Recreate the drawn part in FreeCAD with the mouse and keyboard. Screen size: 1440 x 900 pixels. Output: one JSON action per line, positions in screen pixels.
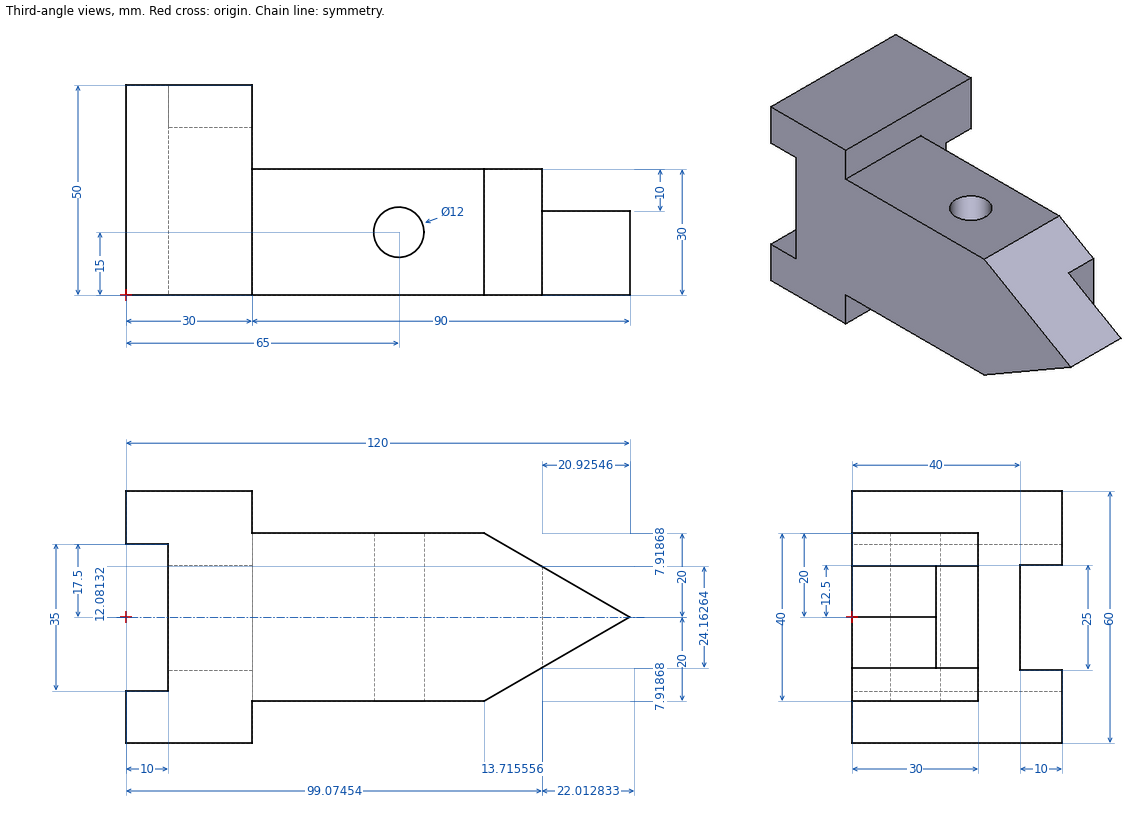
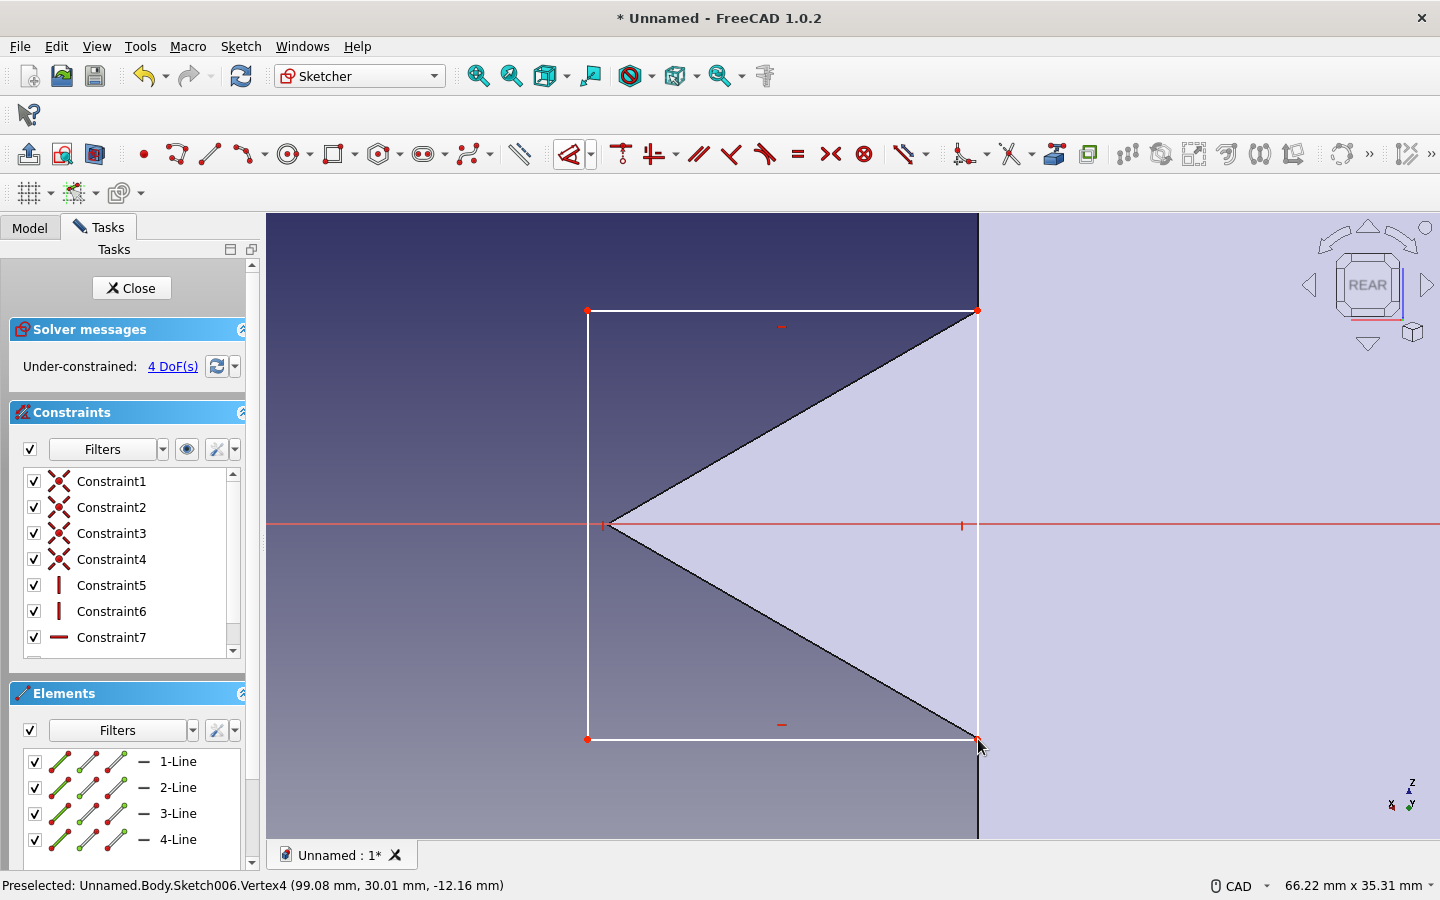
{"action": "left_click", "coordinate": [588, 440]}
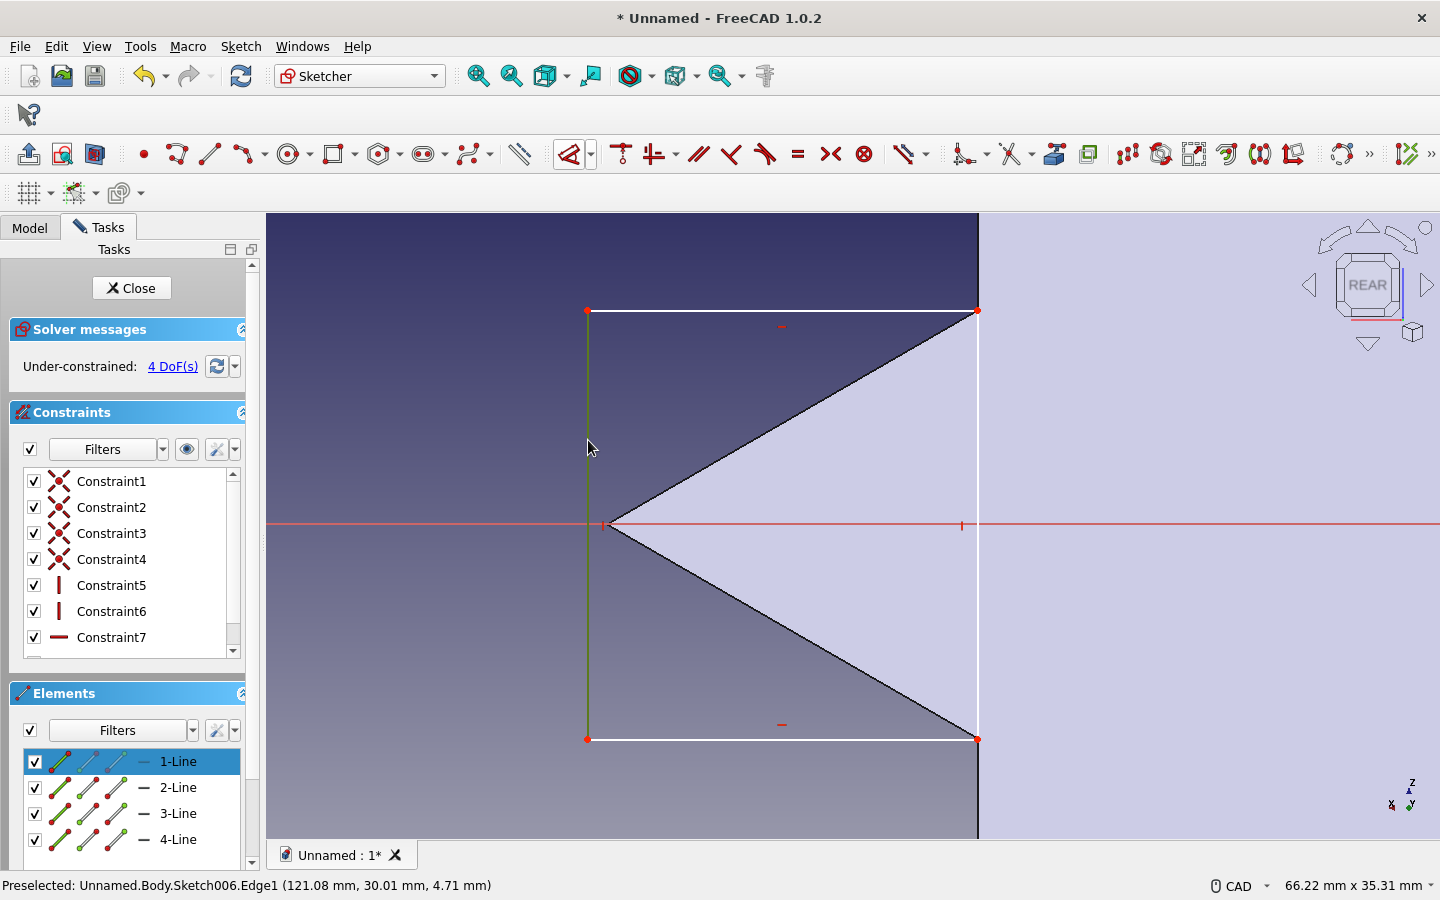
{"action": "left_click", "coordinate": [590, 154]}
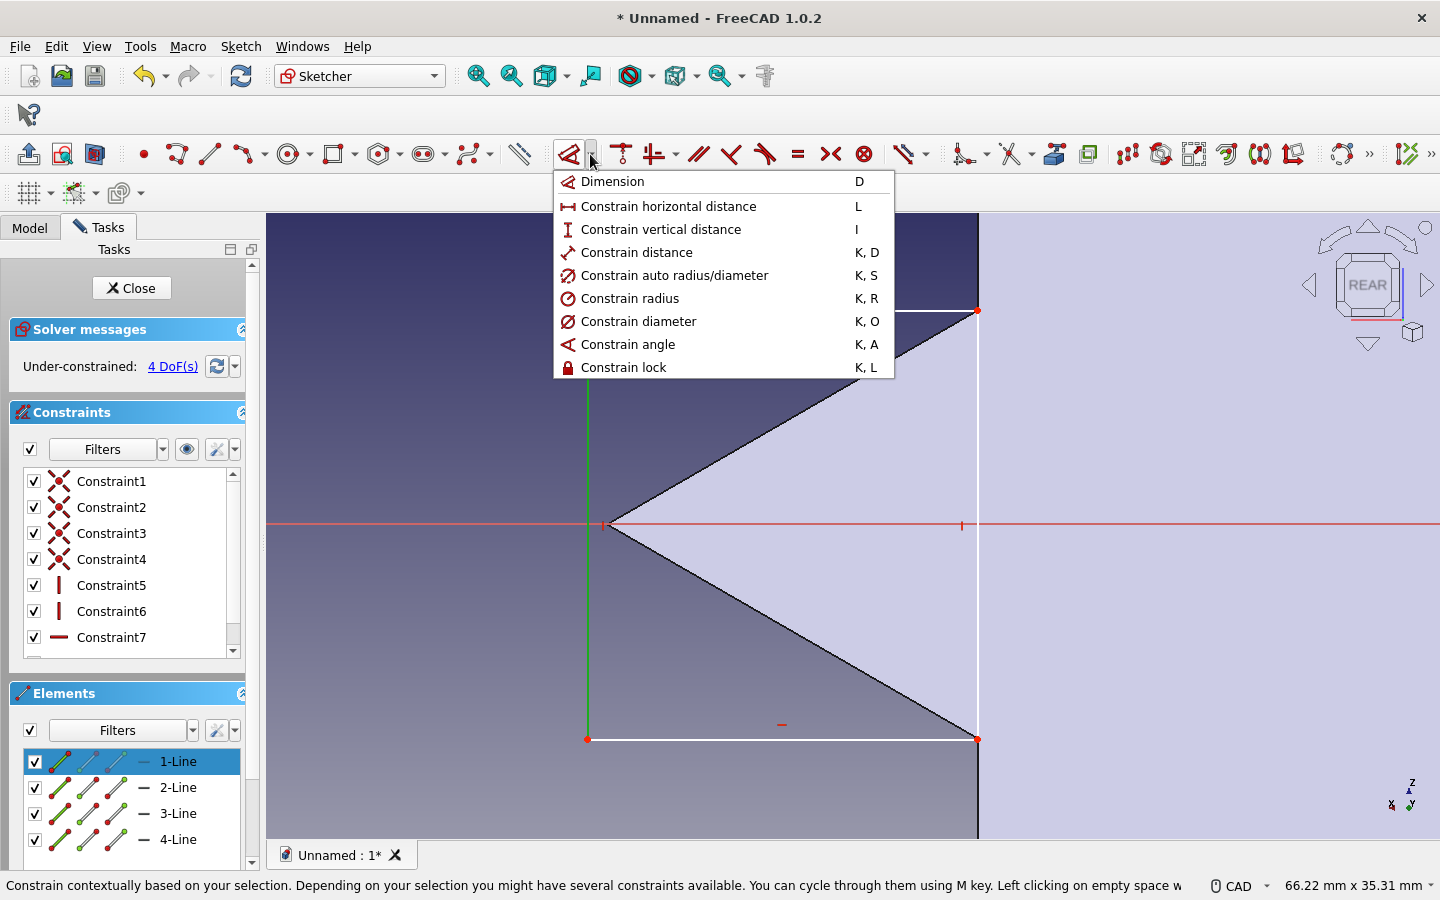
{"action": "left_click", "coordinate": [724, 230]}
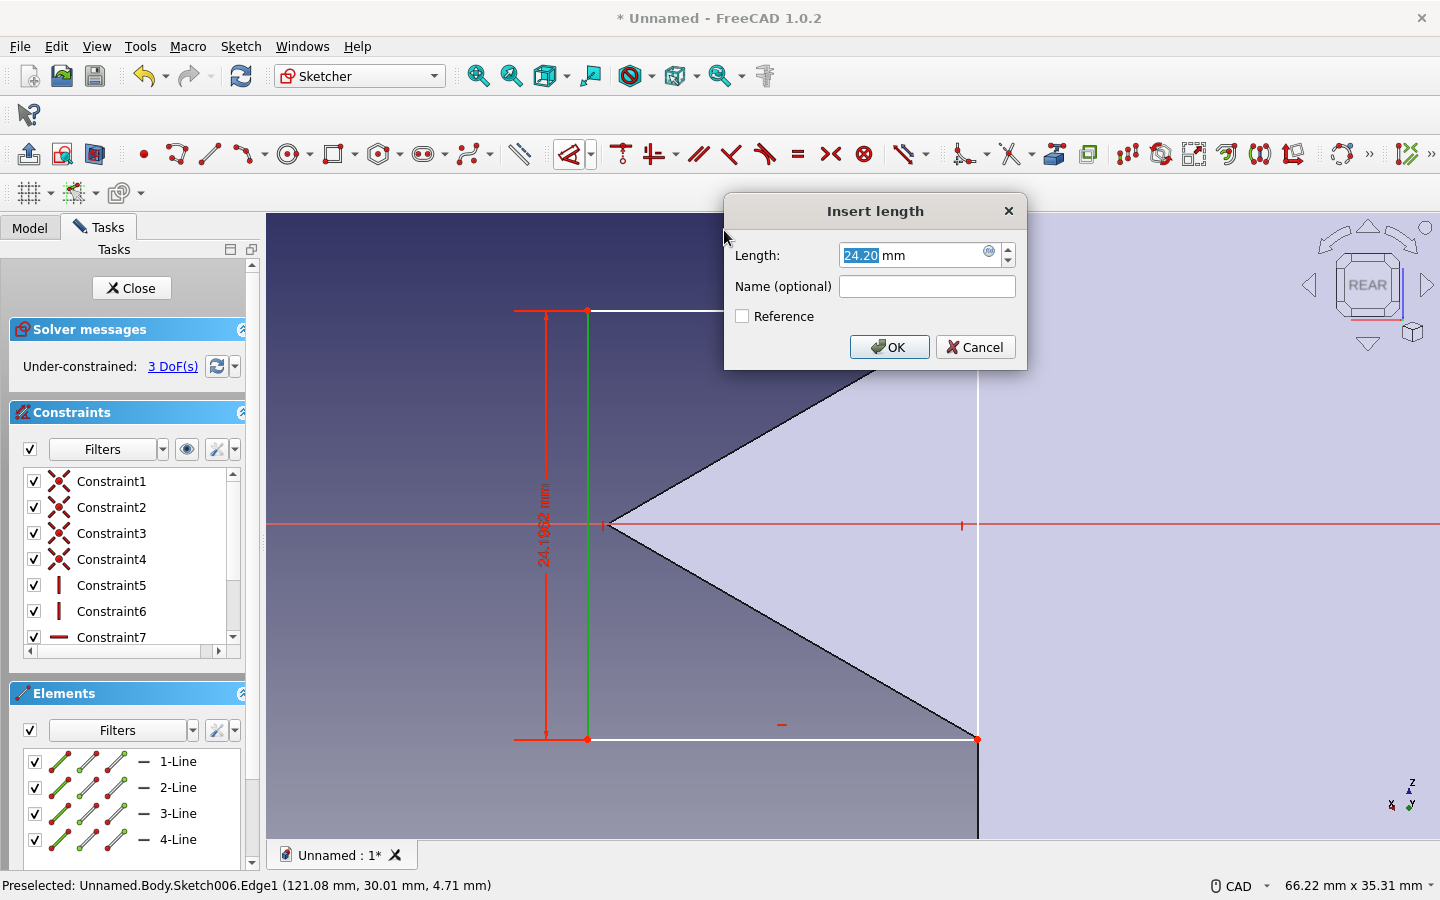
{"action": "type", "text": "24.16264"}
{"action": "key", "text": "Return"}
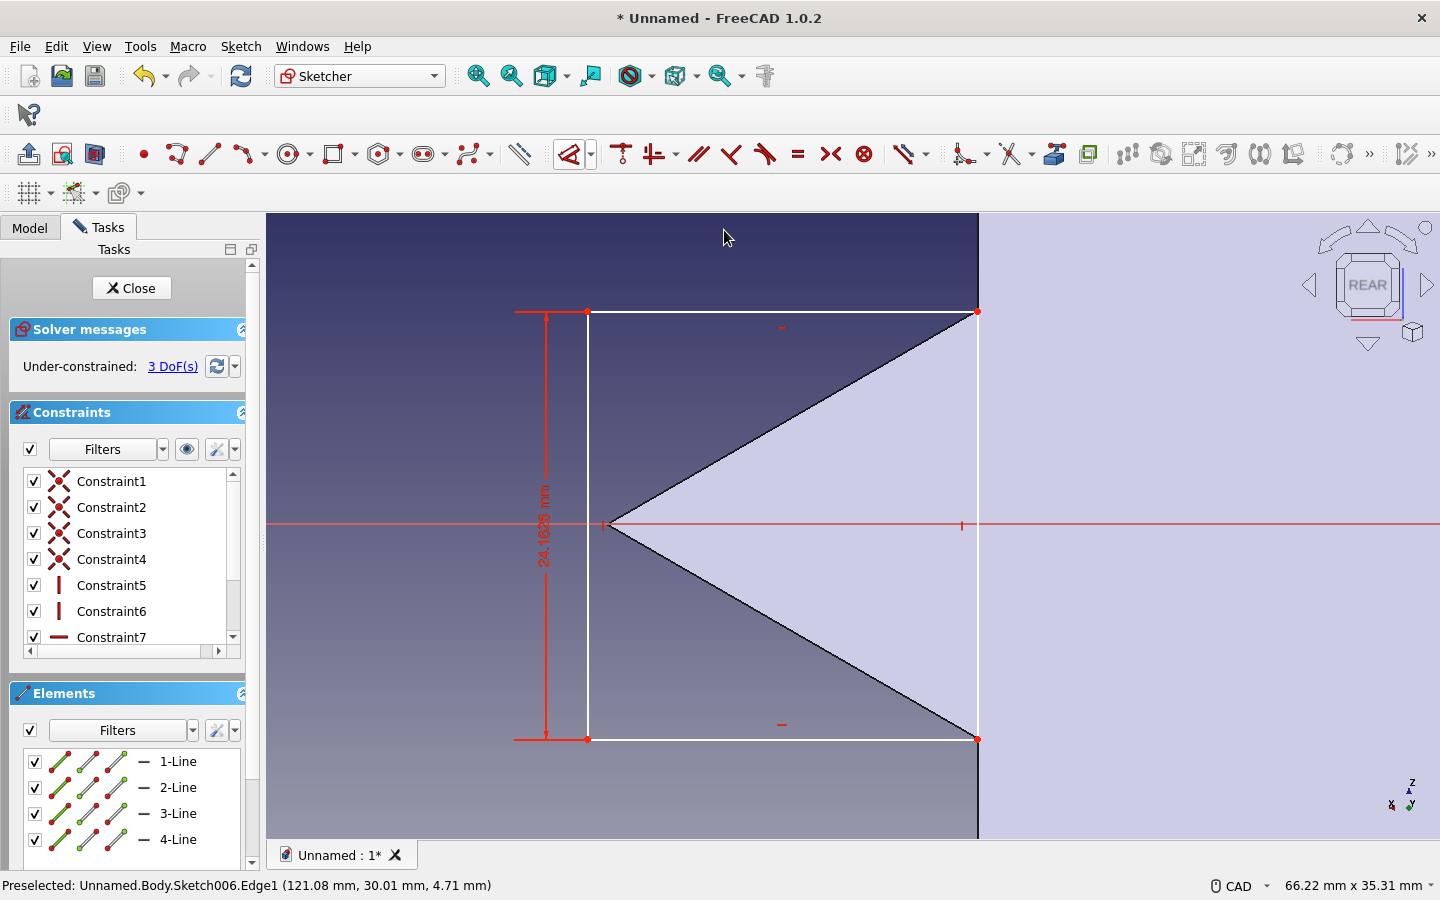
{"action": "left_click", "coordinate": [705, 740]}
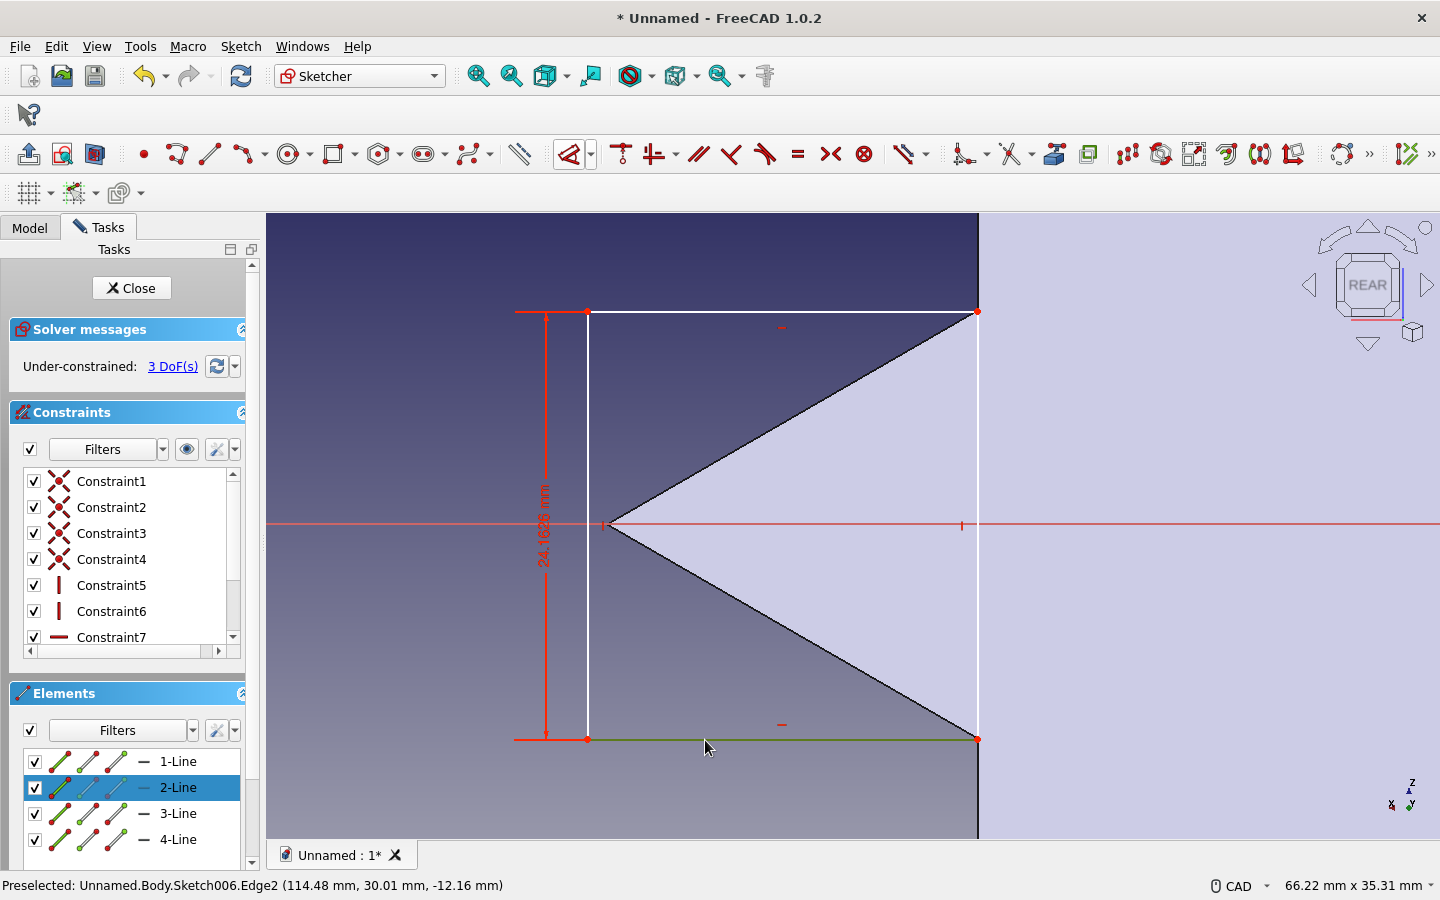
{"action": "left_click", "coordinate": [590, 154]}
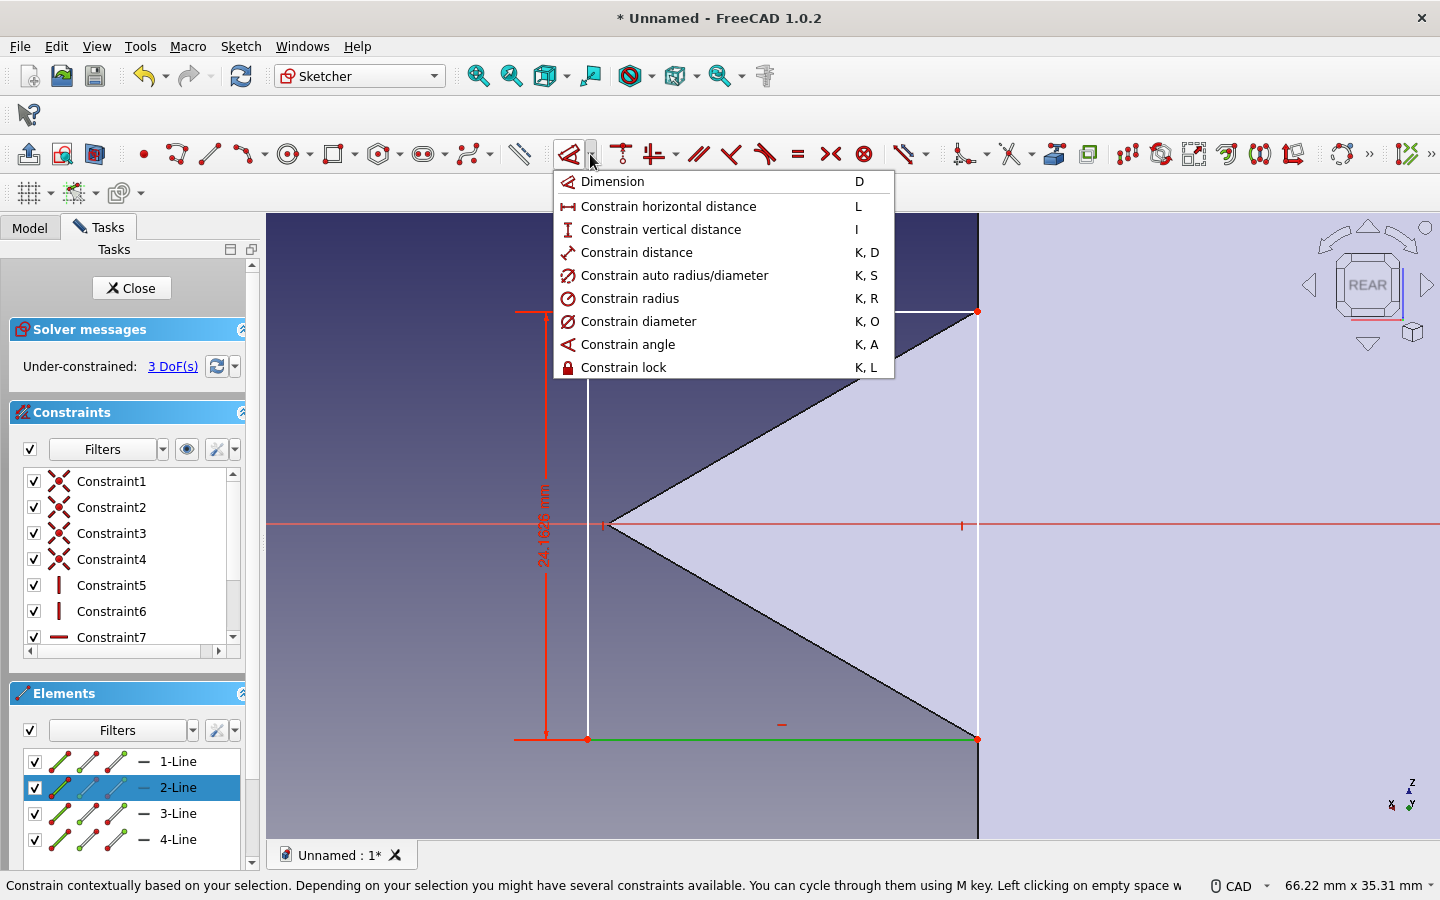
{"action": "left_click", "coordinate": [724, 206]}